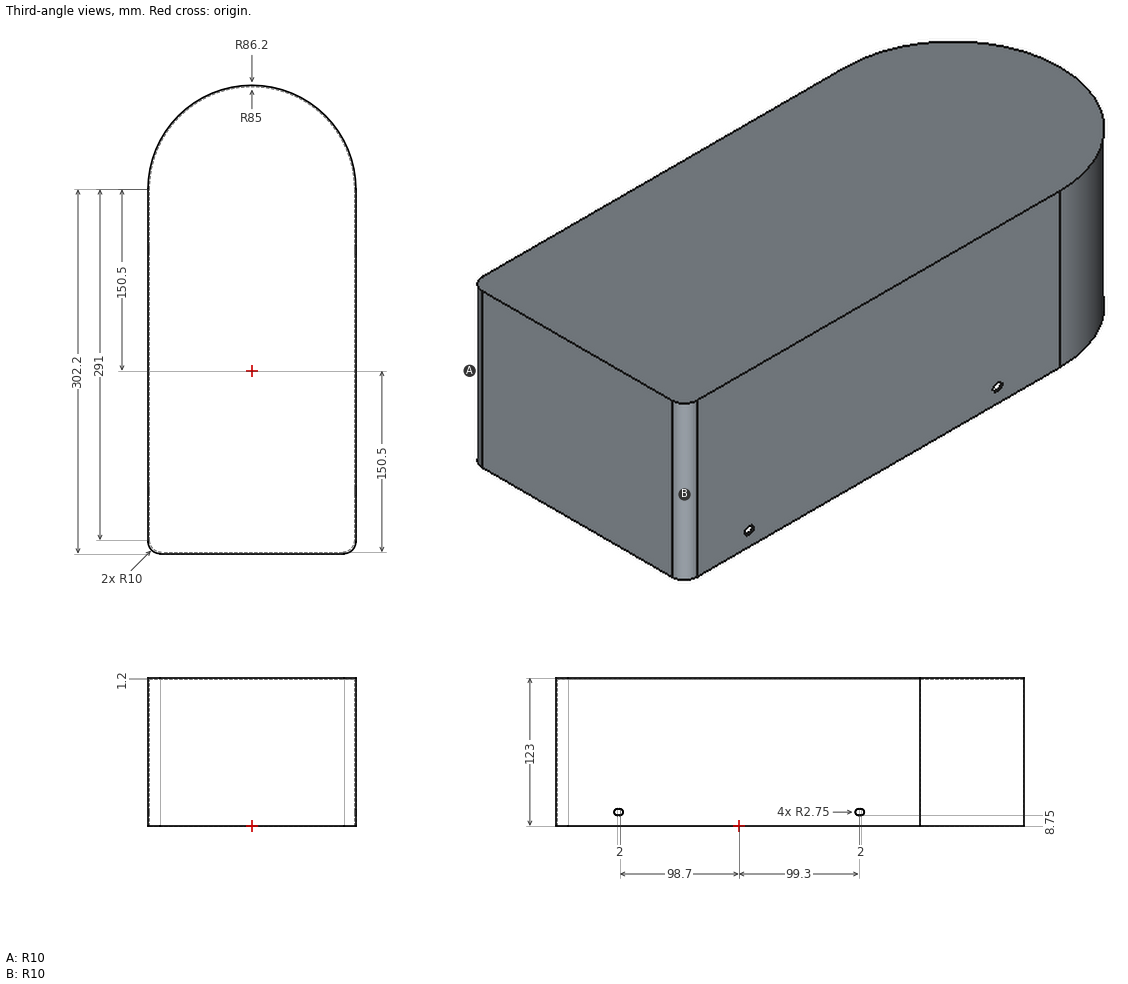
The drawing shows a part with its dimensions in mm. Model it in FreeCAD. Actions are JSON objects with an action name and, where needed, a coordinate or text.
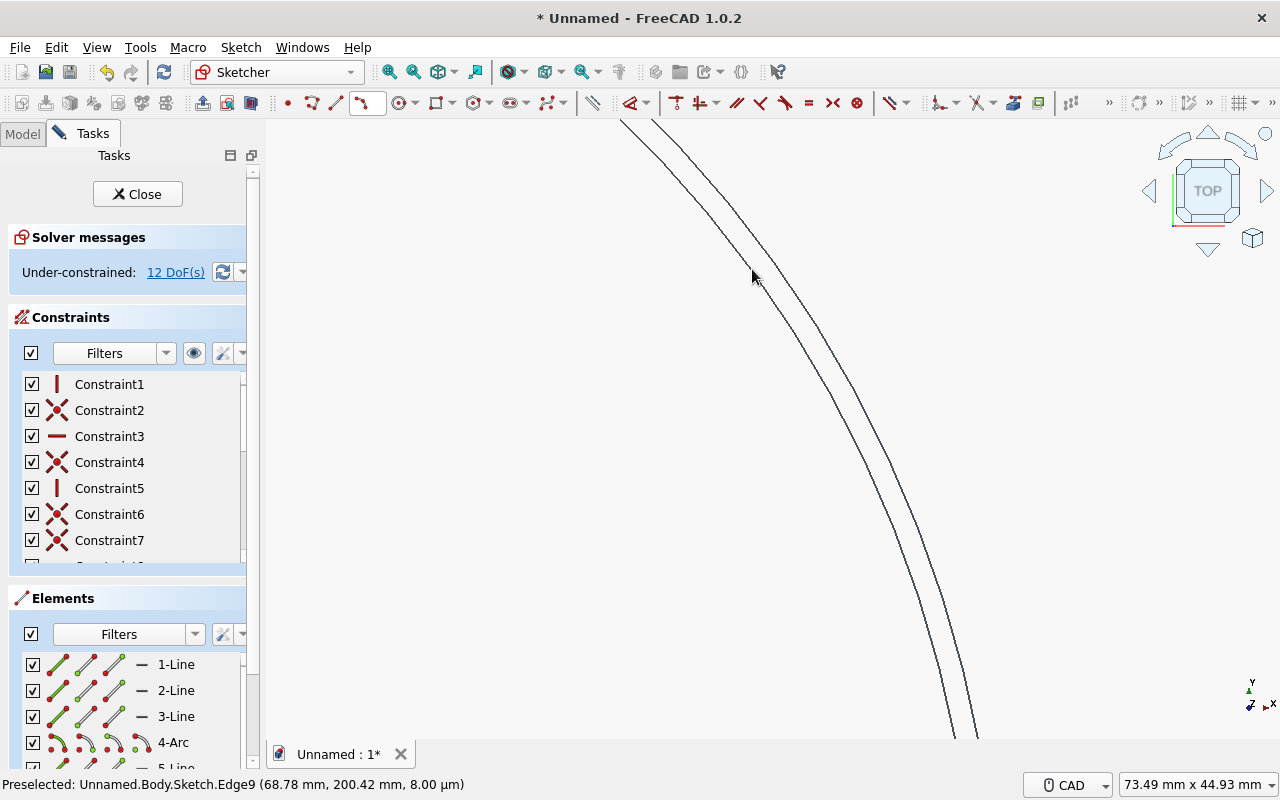
{"action": "scroll", "coordinate": [777, 267], "scroll_direction": "down", "scroll_amount": 13}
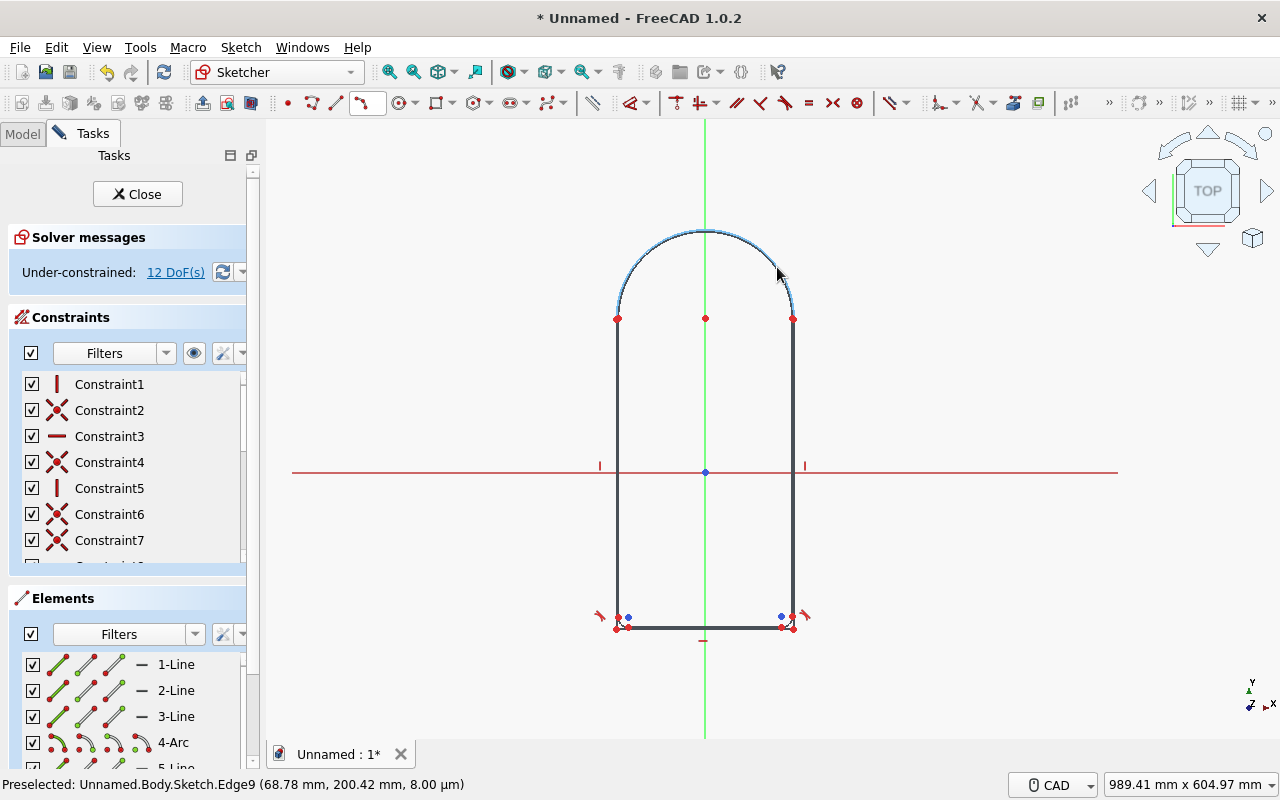
{"action": "scroll", "coordinate": [619, 622], "scroll_direction": "up", "scroll_amount": 9}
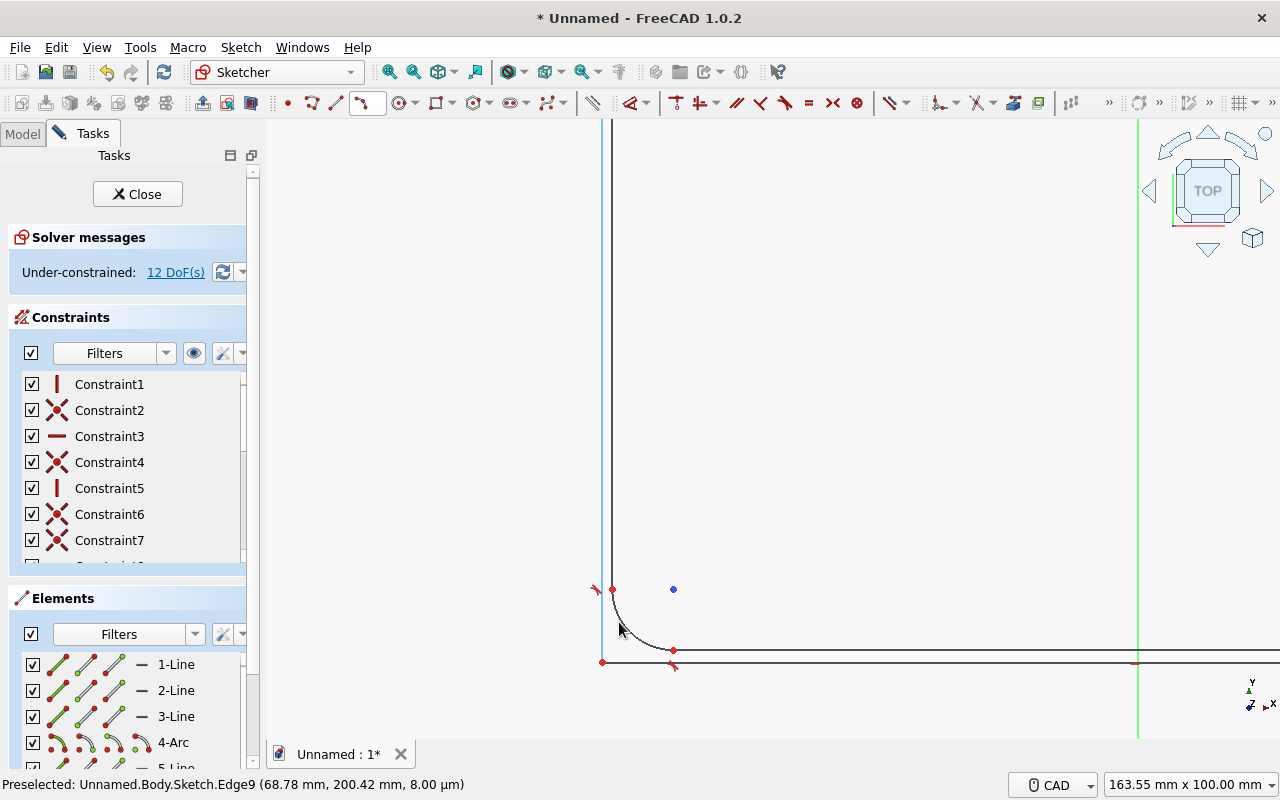
{"action": "left_click", "coordinate": [619, 617]}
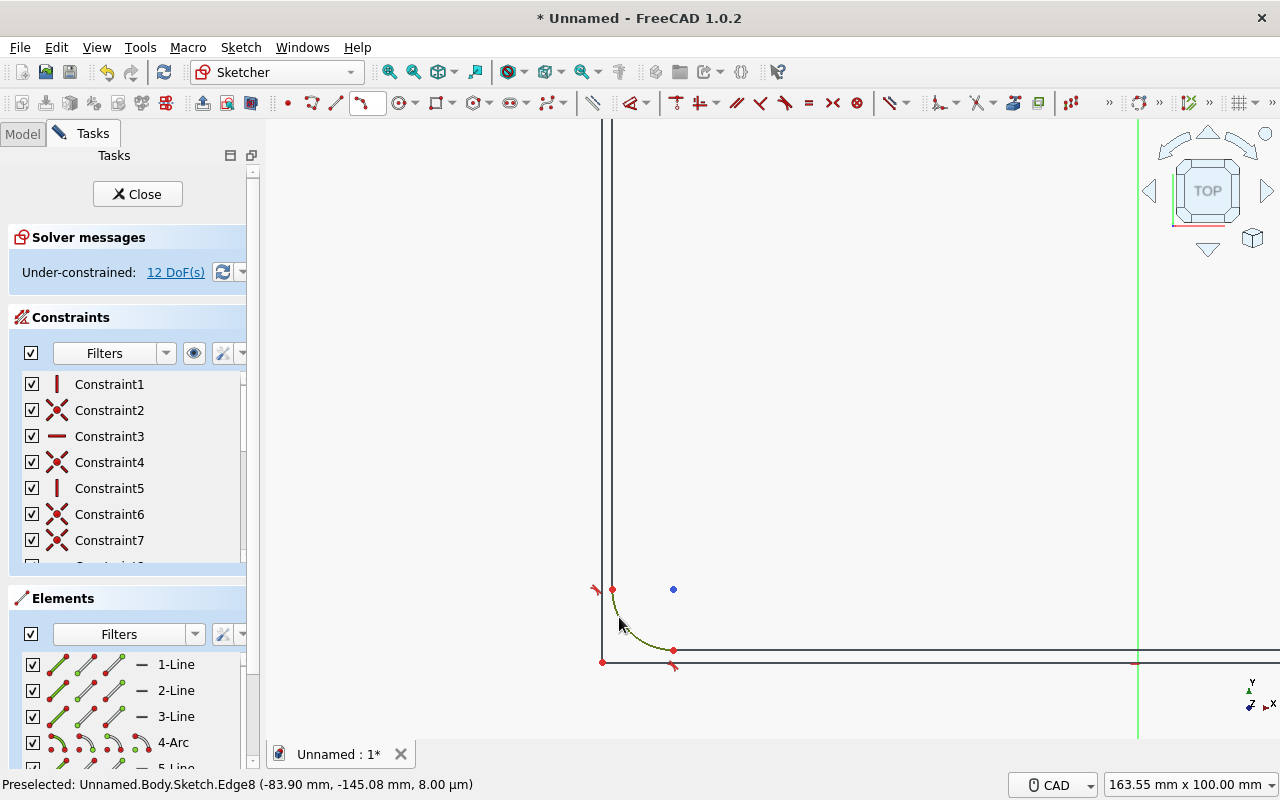
{"action": "scroll", "coordinate": [619, 622], "scroll_direction": "down", "scroll_amount": 9}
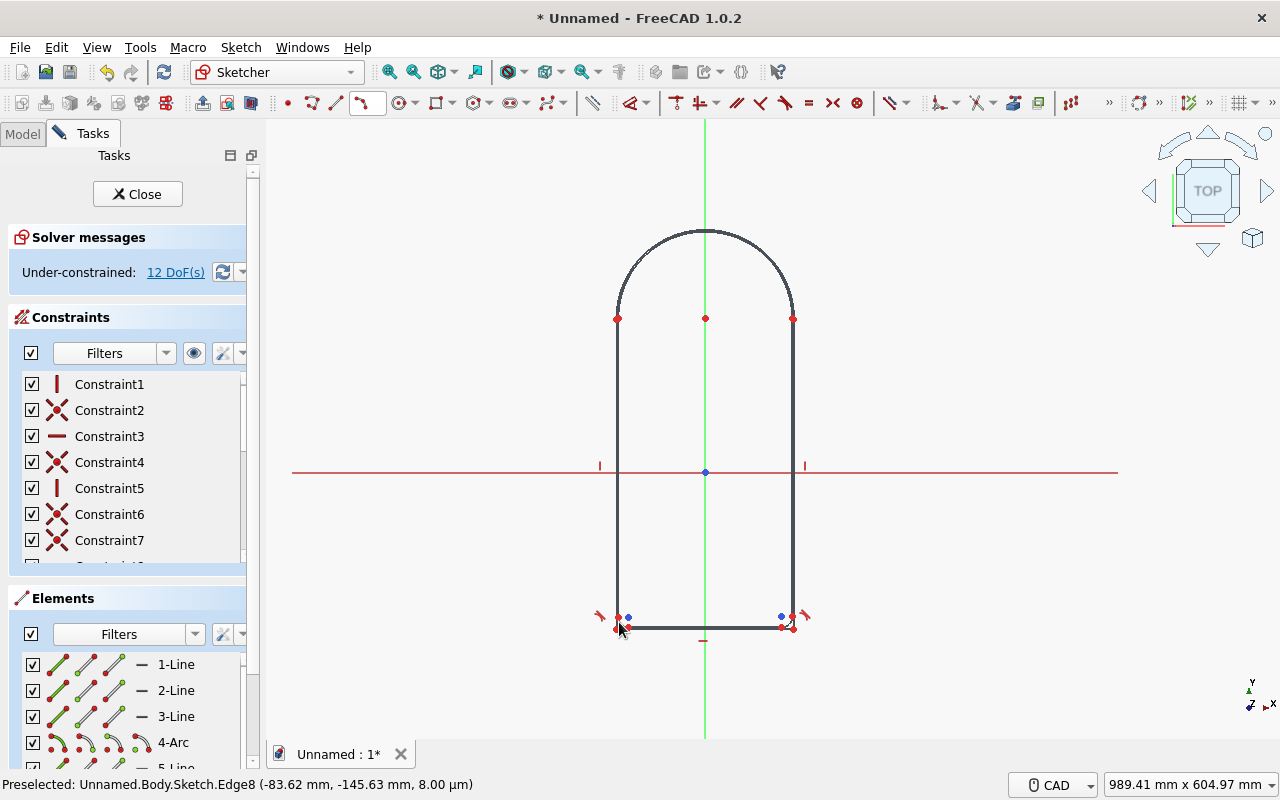
{"action": "scroll", "coordinate": [787, 626], "scroll_direction": "up", "scroll_amount": 8}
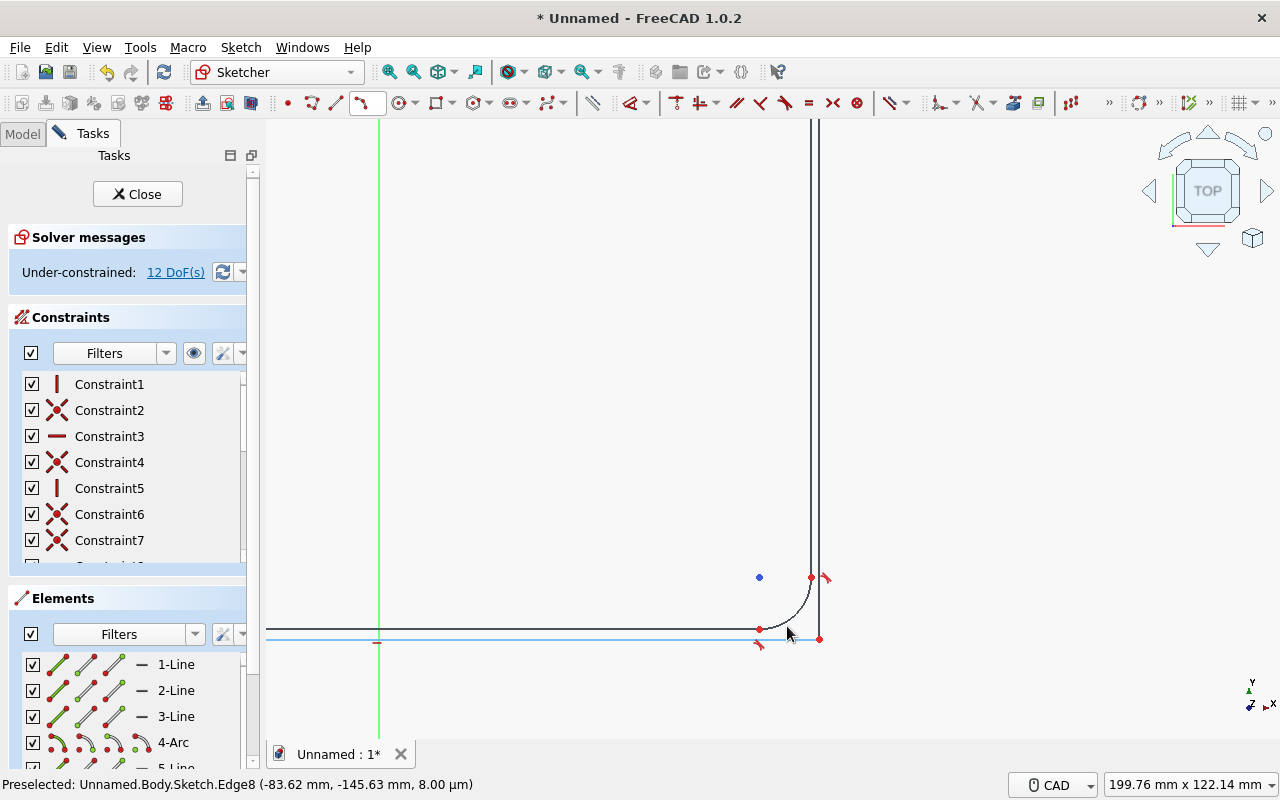
{"action": "left_click", "coordinate": [783, 624]}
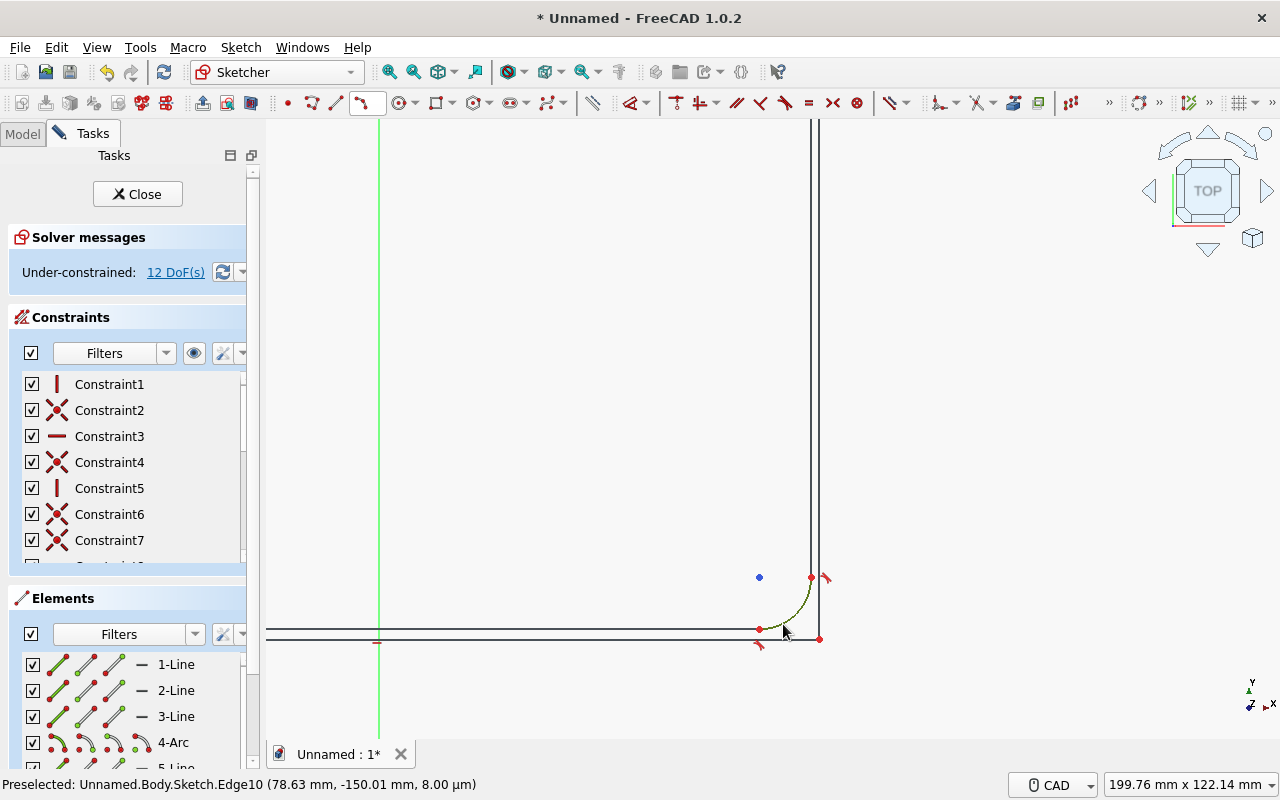
{"action": "key", "text": "e"}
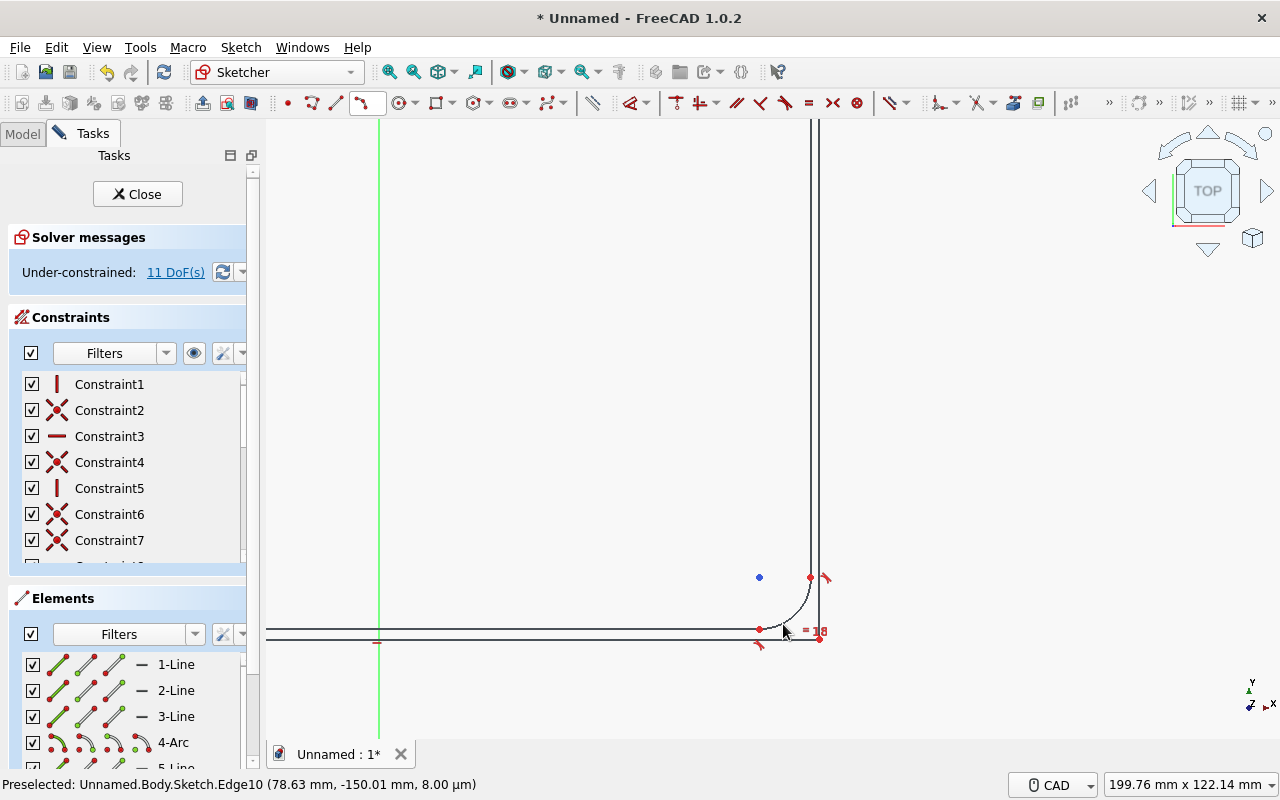
{"action": "scroll", "coordinate": [787, 626], "scroll_direction": "down", "scroll_amount": 8}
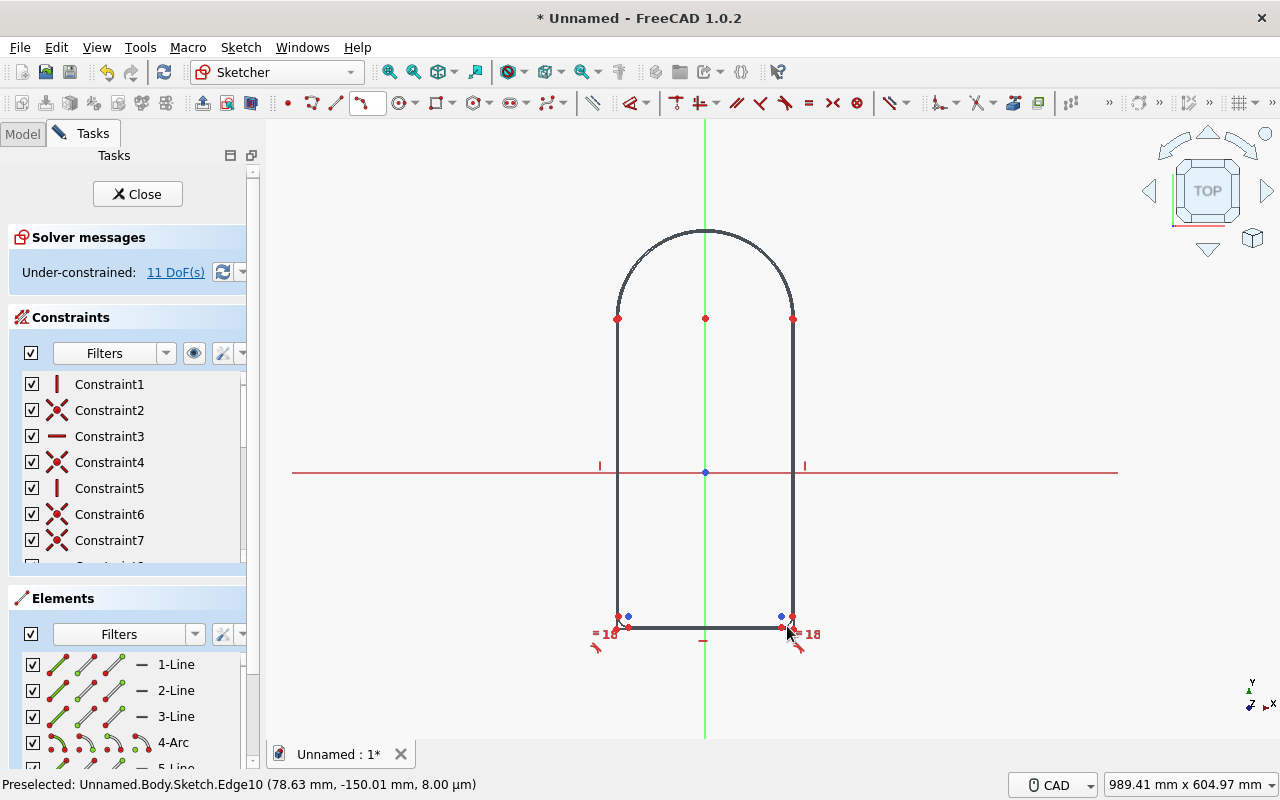
{"action": "left_click", "coordinate": [705, 319]}